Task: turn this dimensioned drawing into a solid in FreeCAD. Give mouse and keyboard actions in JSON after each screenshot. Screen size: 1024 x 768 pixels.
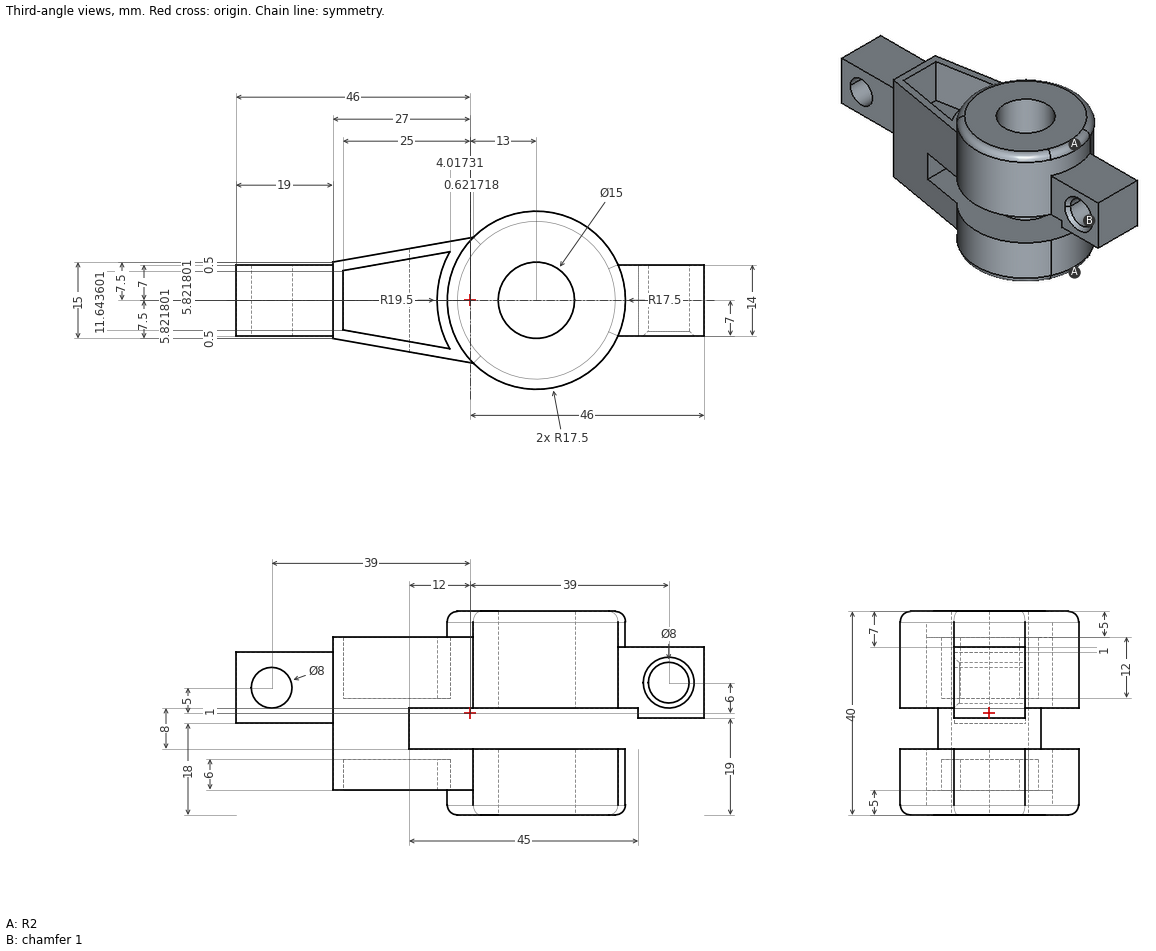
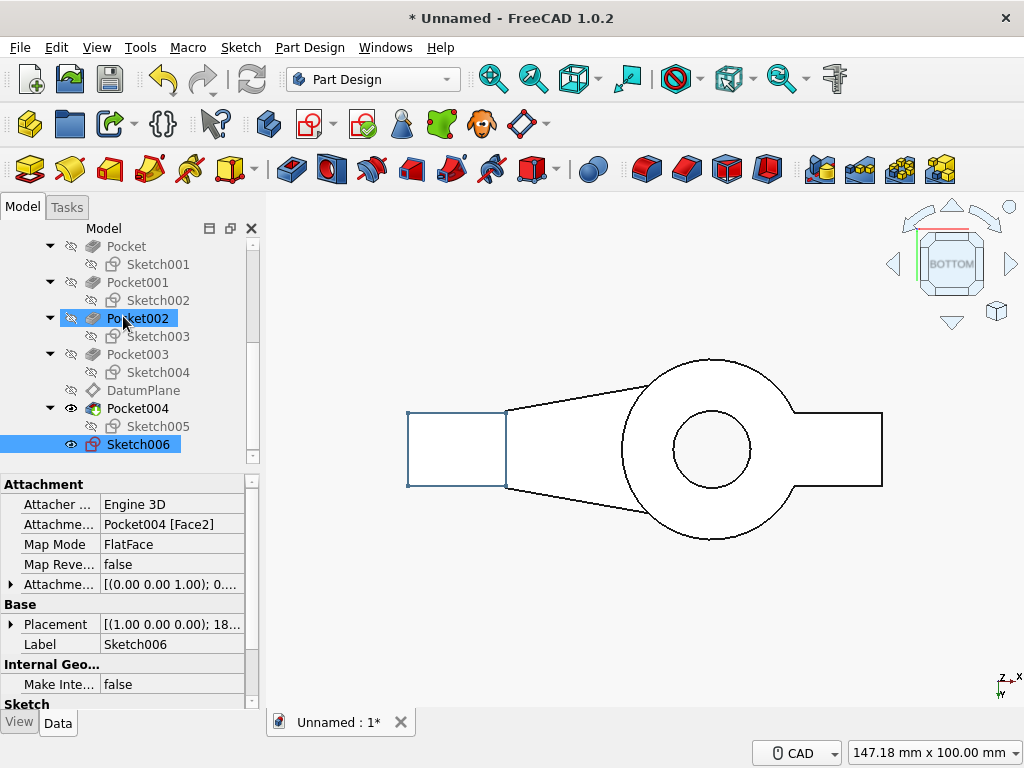
{"action": "left_click", "coordinate": [292, 170]}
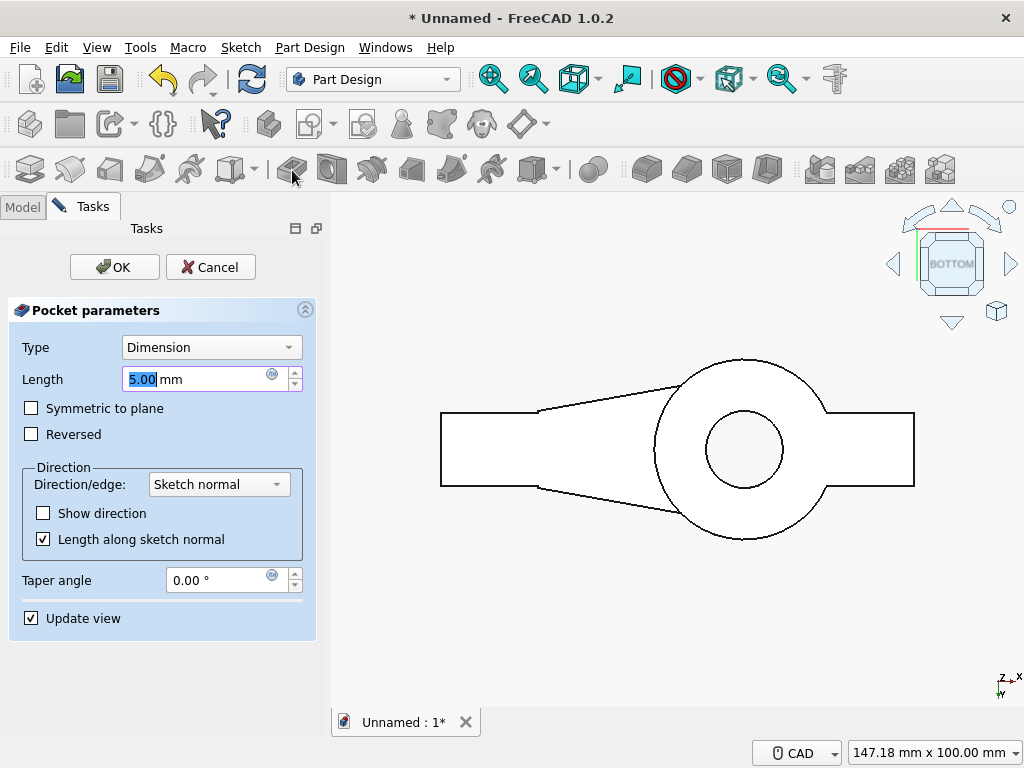
{"action": "type", "text": "18"}
{"action": "key", "text": "Tab"}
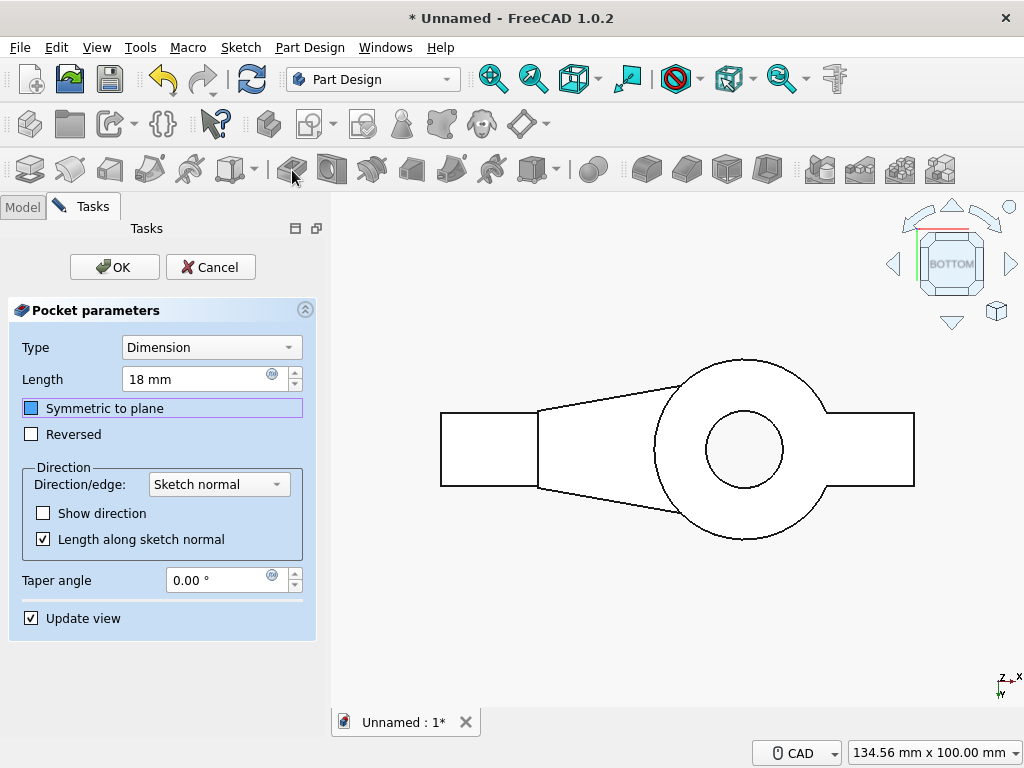
{"action": "left_click", "coordinate": [115, 267]}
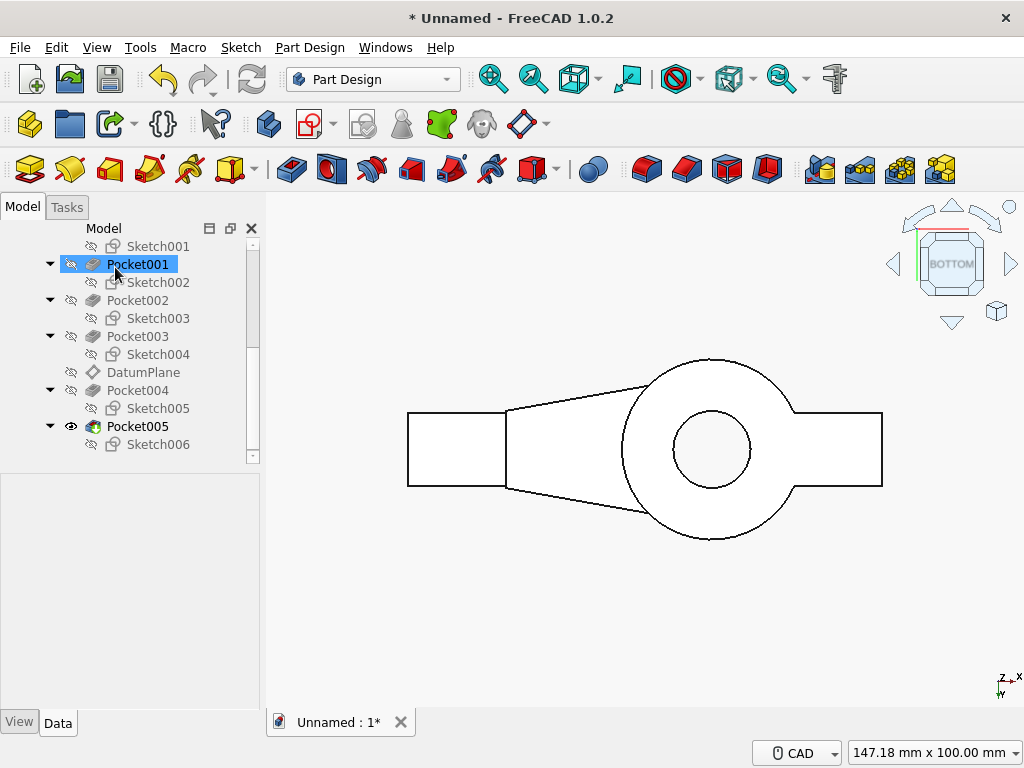
{"action": "key", "text": "0"}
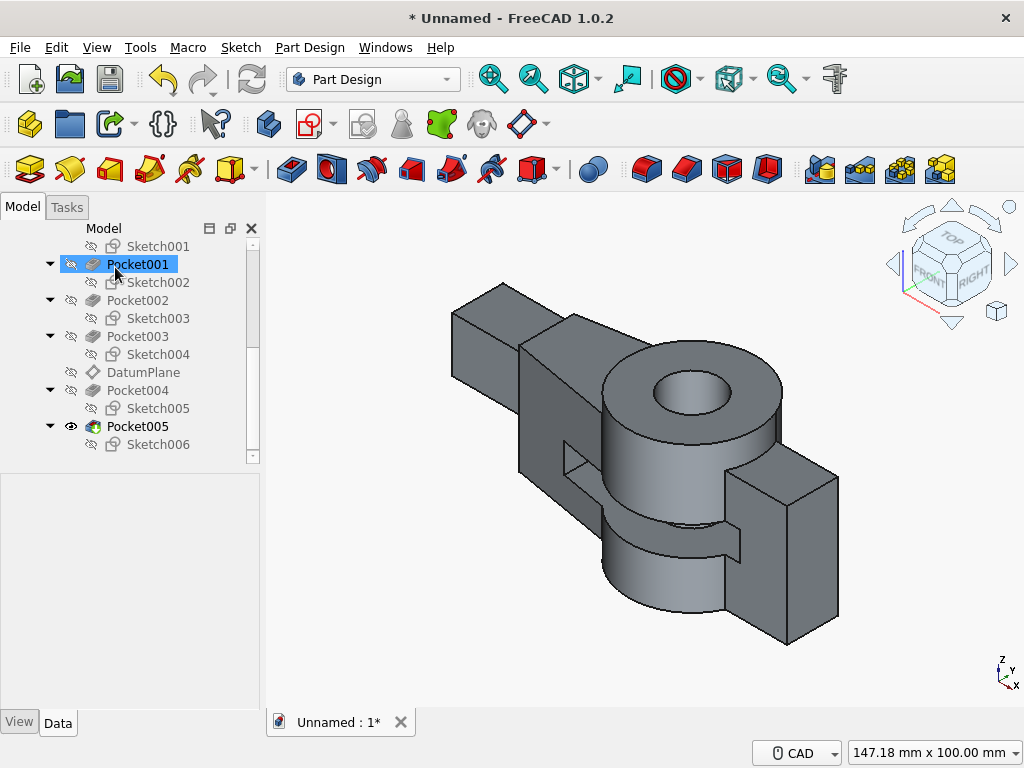
{"action": "left_click", "coordinate": [512, 317]}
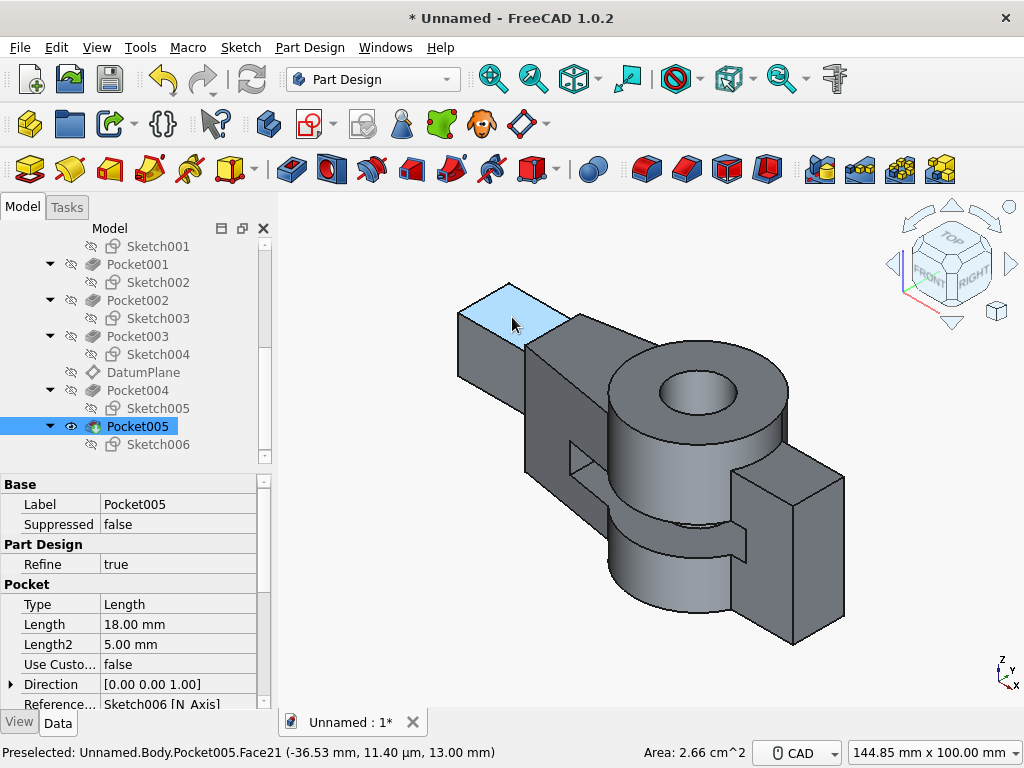
{"action": "left_click", "coordinate": [310, 124]}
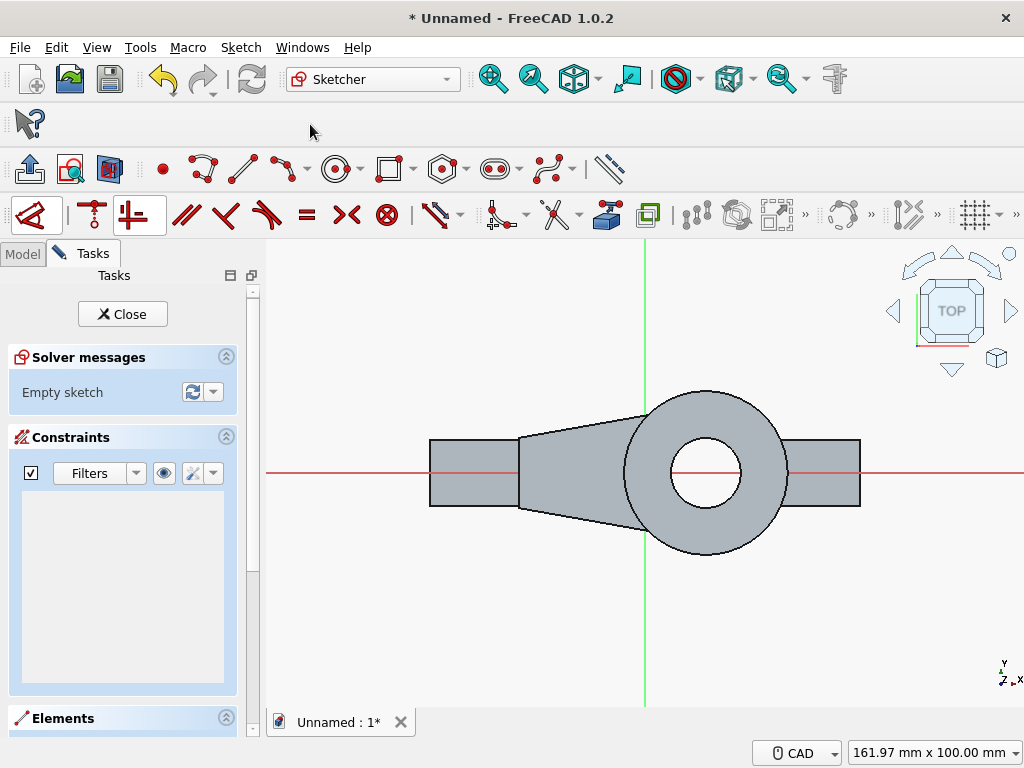
{"action": "left_click", "coordinate": [110, 170]}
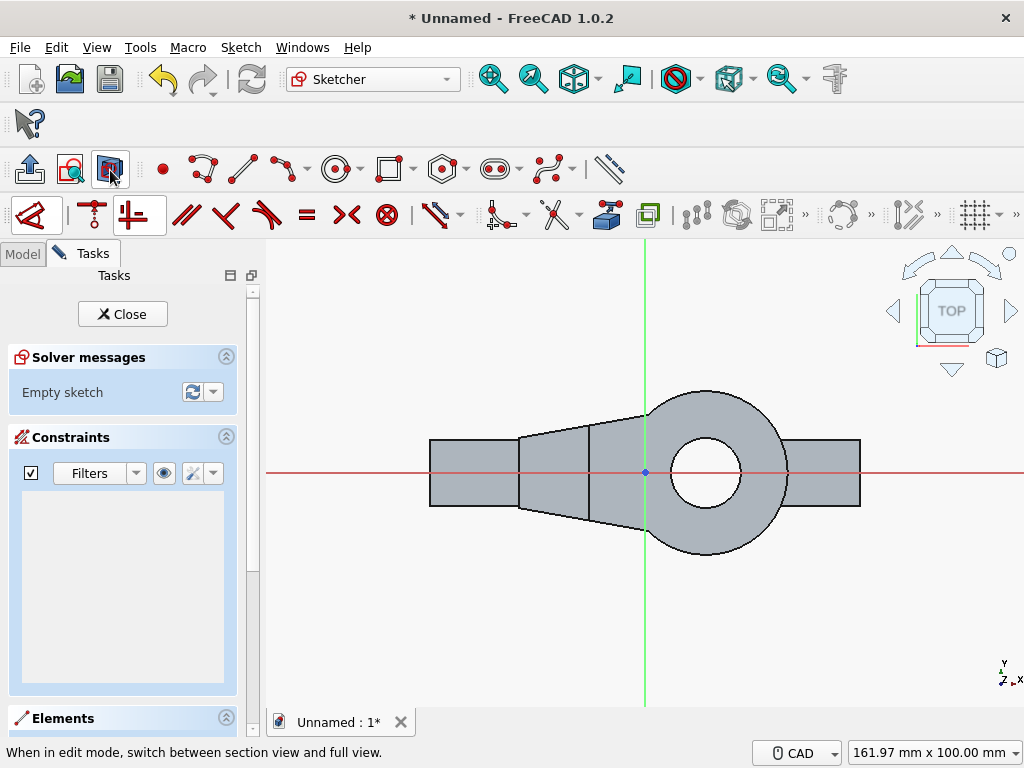
{"action": "scroll", "coordinate": [490, 473], "scroll_direction": "up", "scroll_amount": 3}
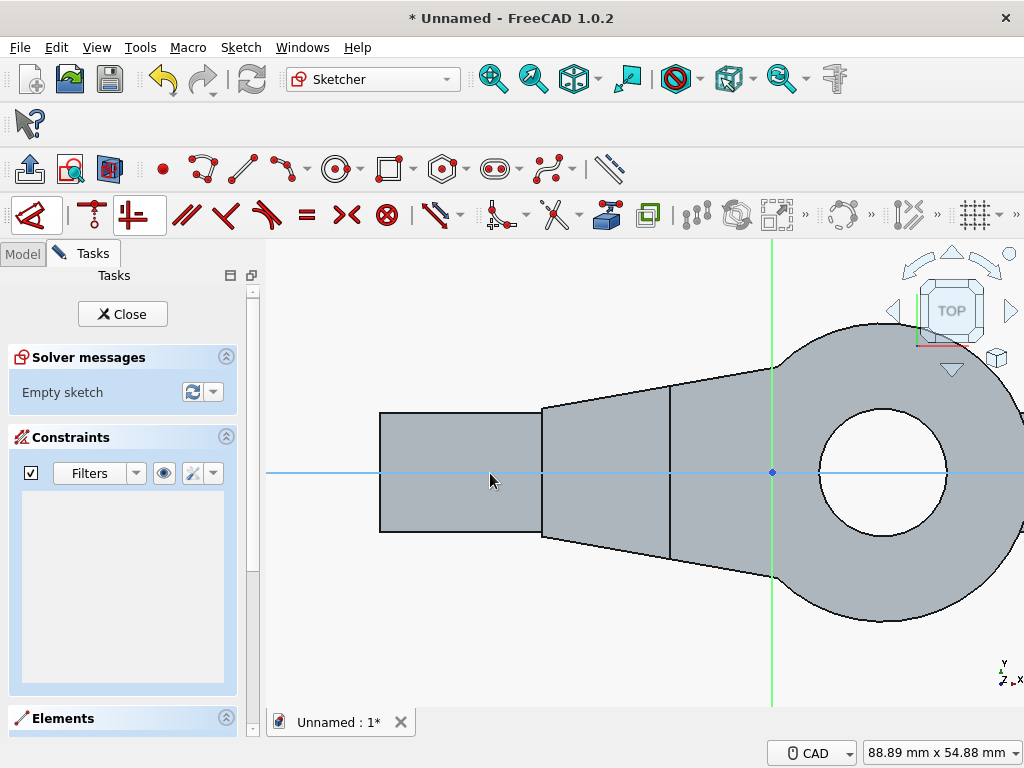
{"action": "left_click", "coordinate": [390, 170]}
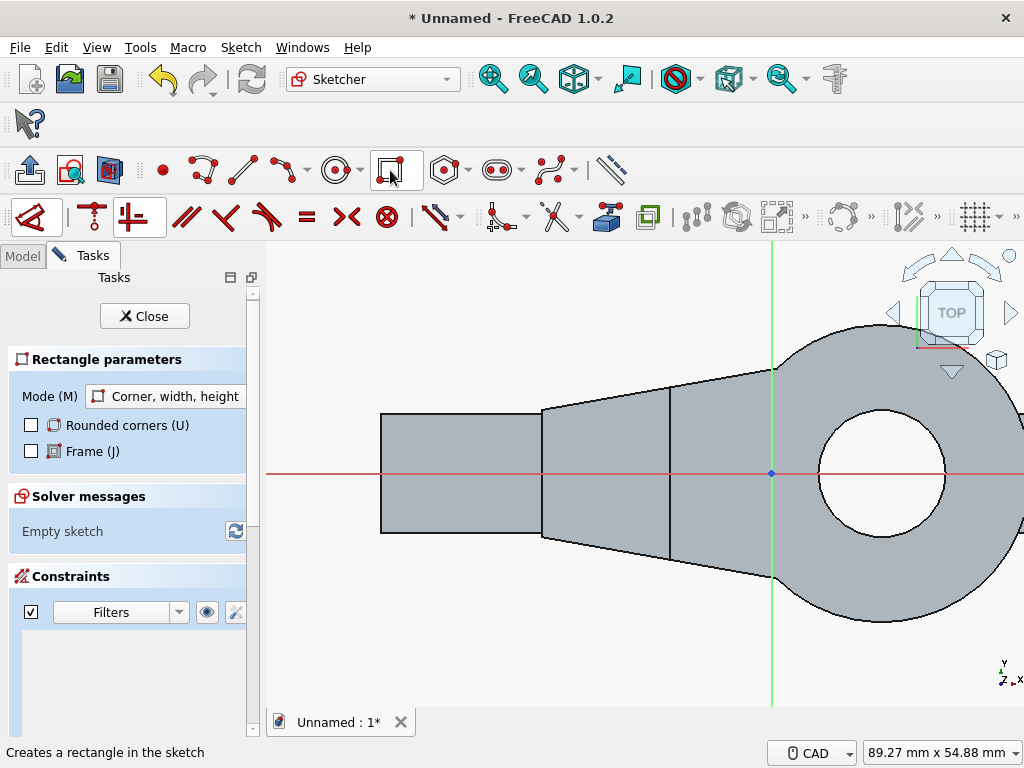
{"action": "left_click", "coordinate": [381, 414]}
{"action": "left_click", "coordinate": [542, 533]}
{"action": "key", "text": "Escape"}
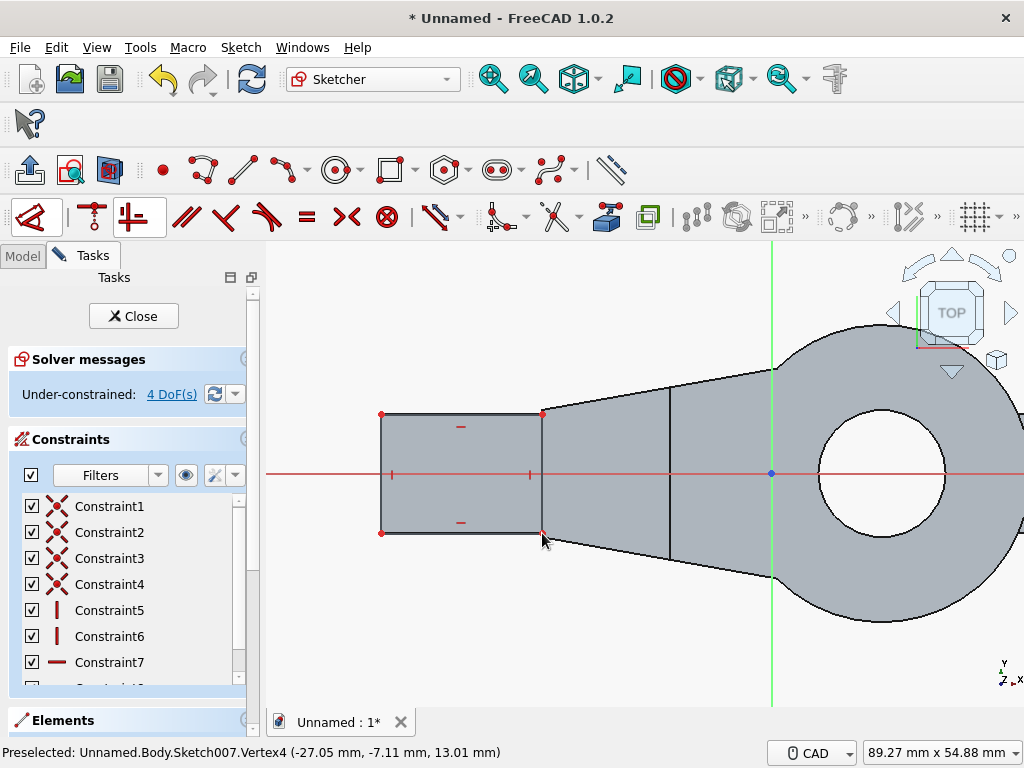
{"action": "left_click", "coordinate": [381, 451]}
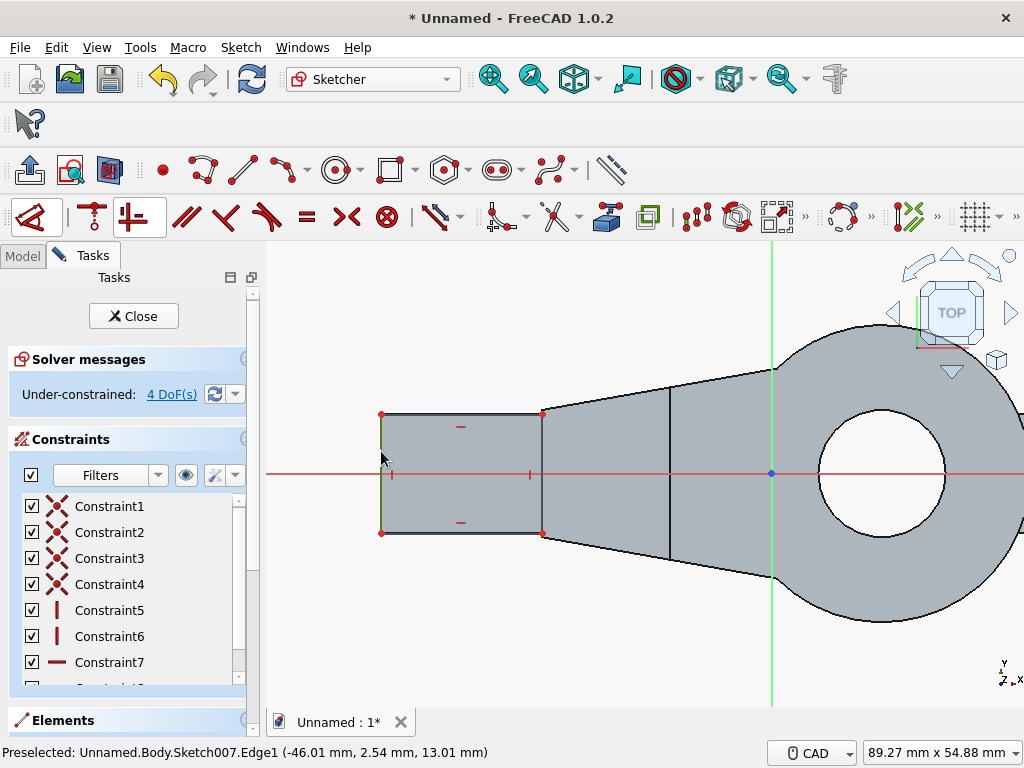
{"action": "left_click", "coordinate": [56, 218]}